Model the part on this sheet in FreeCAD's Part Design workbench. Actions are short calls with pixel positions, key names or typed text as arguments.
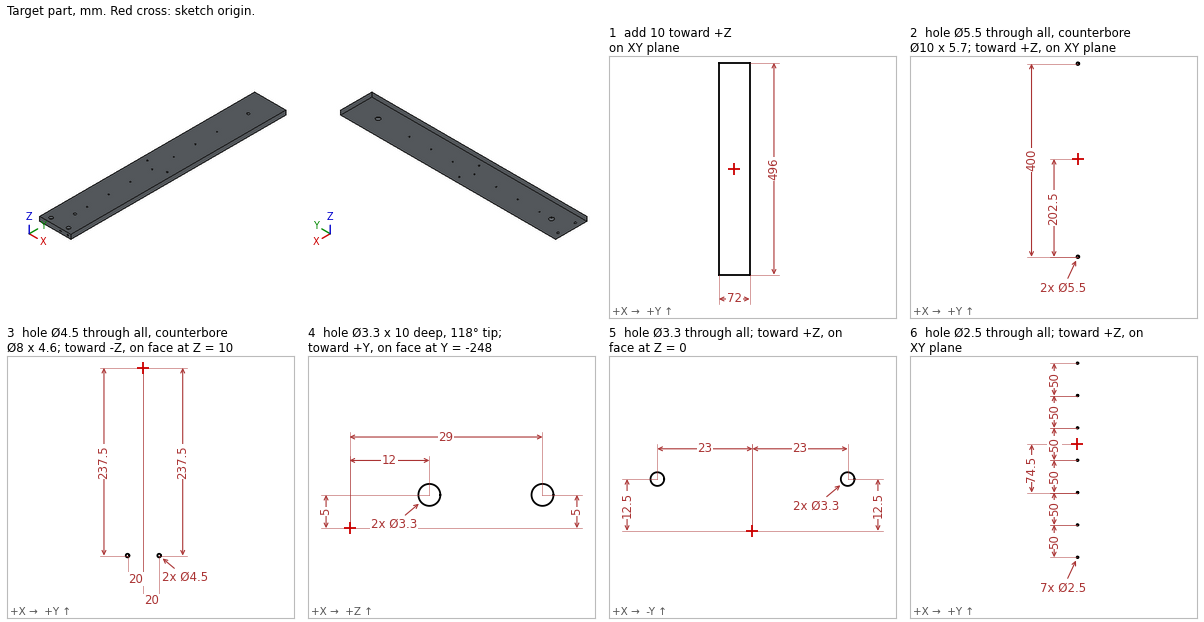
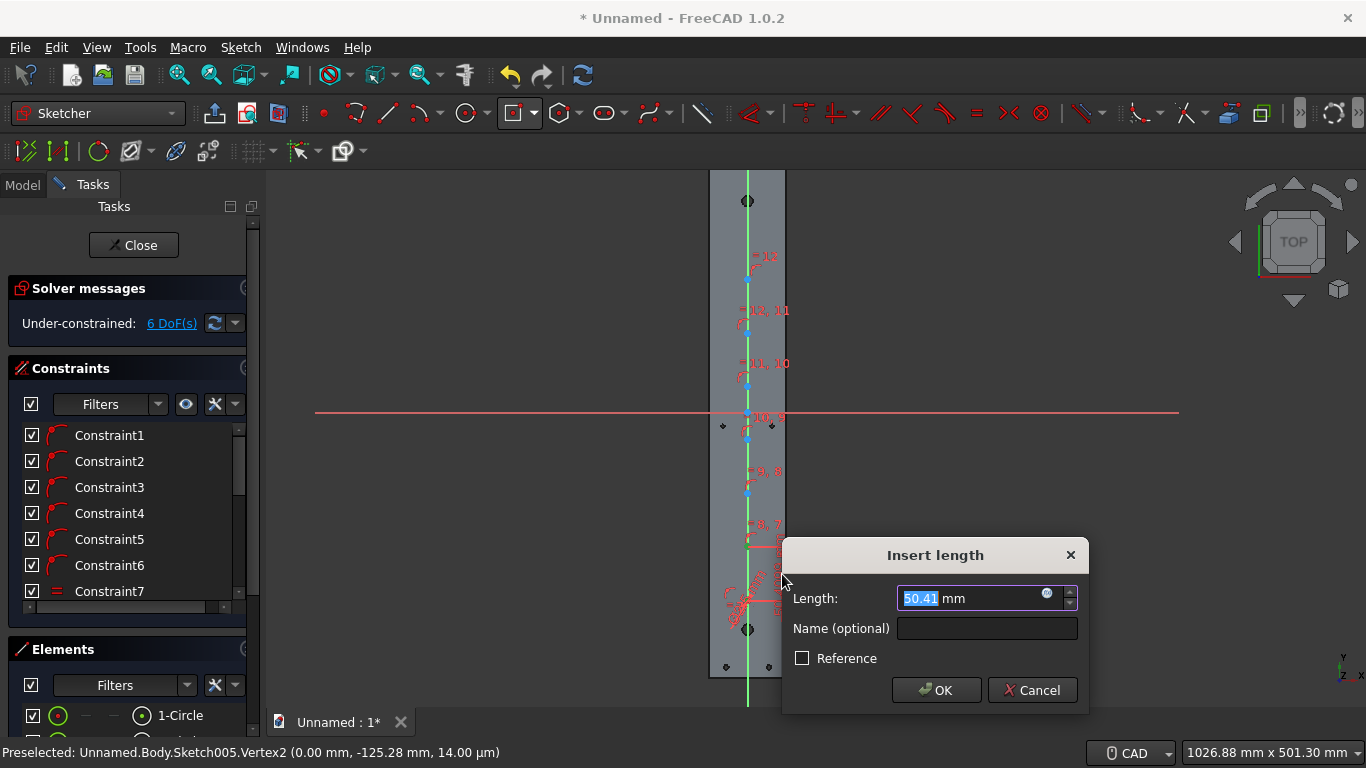
text(50)
key(Return)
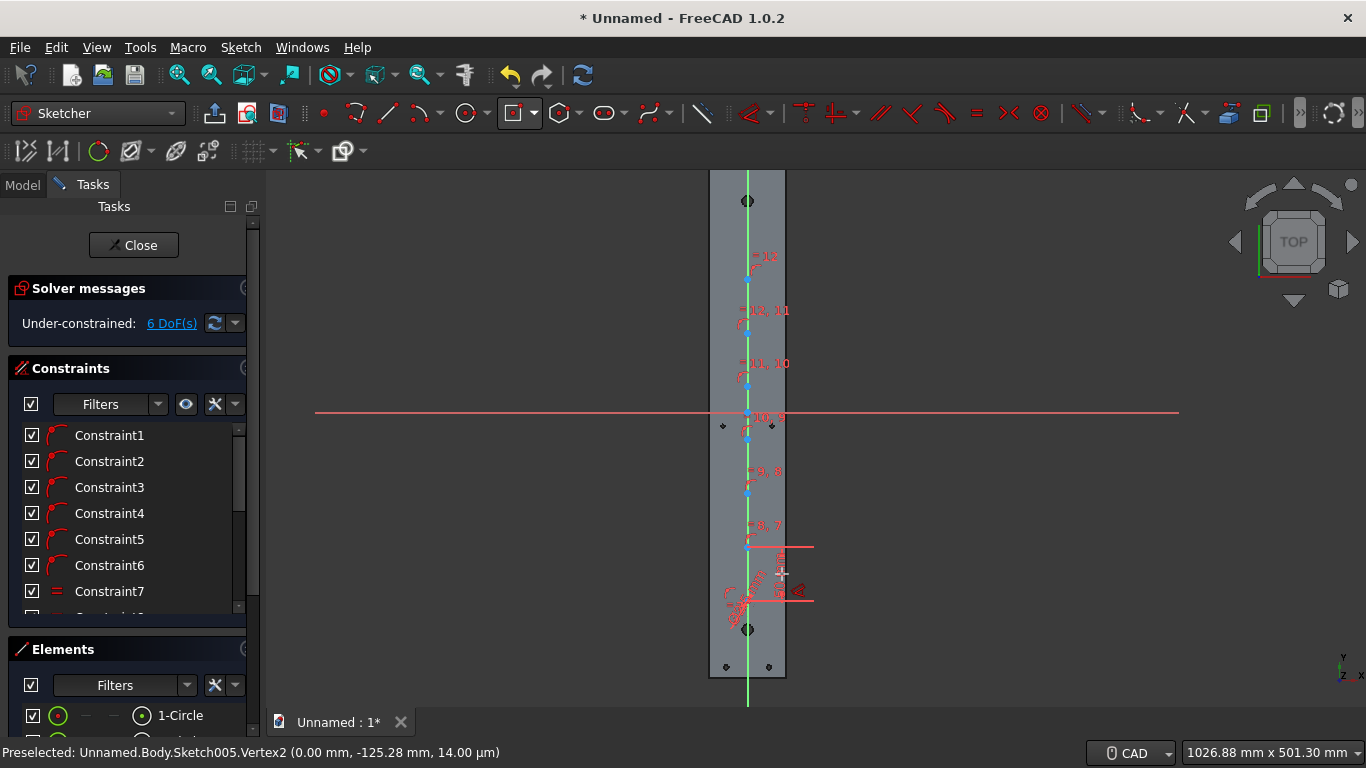
click(748, 547)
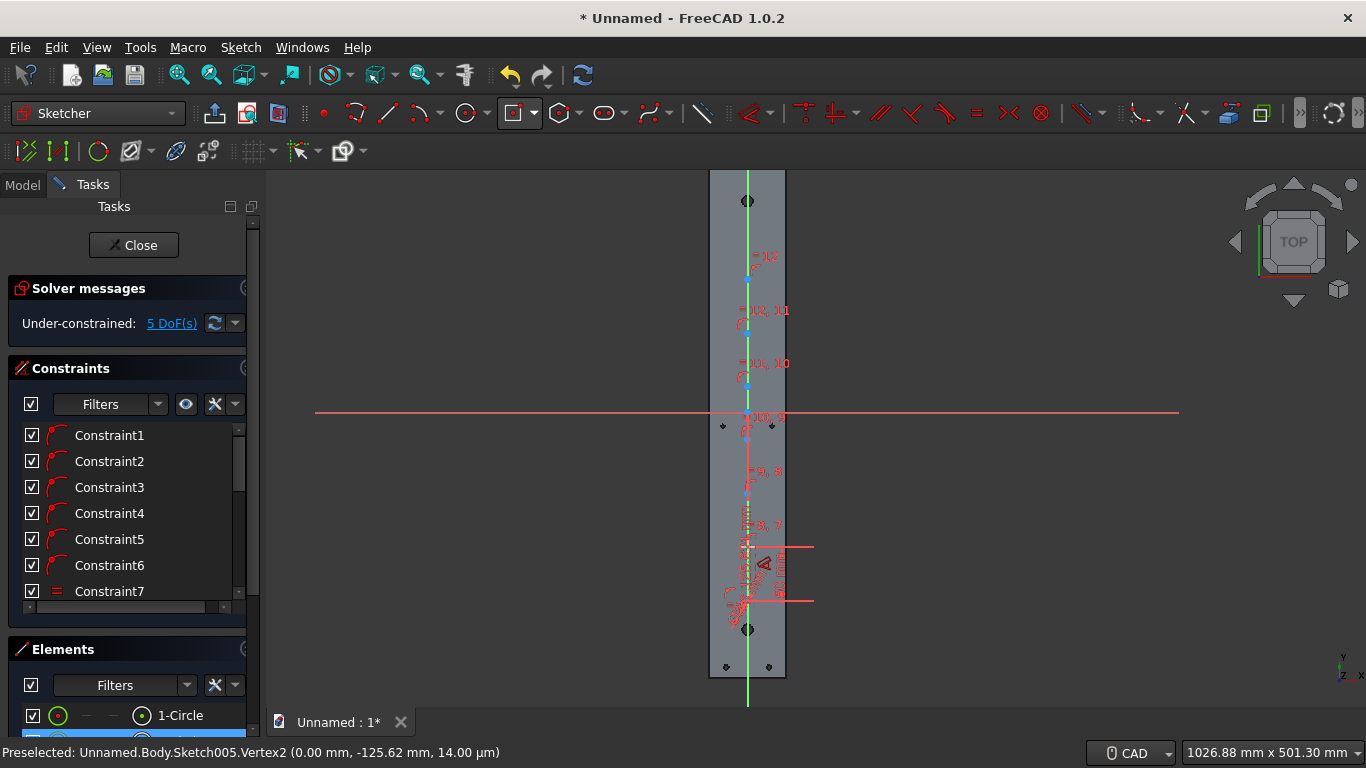
click(748, 494)
click(782, 521)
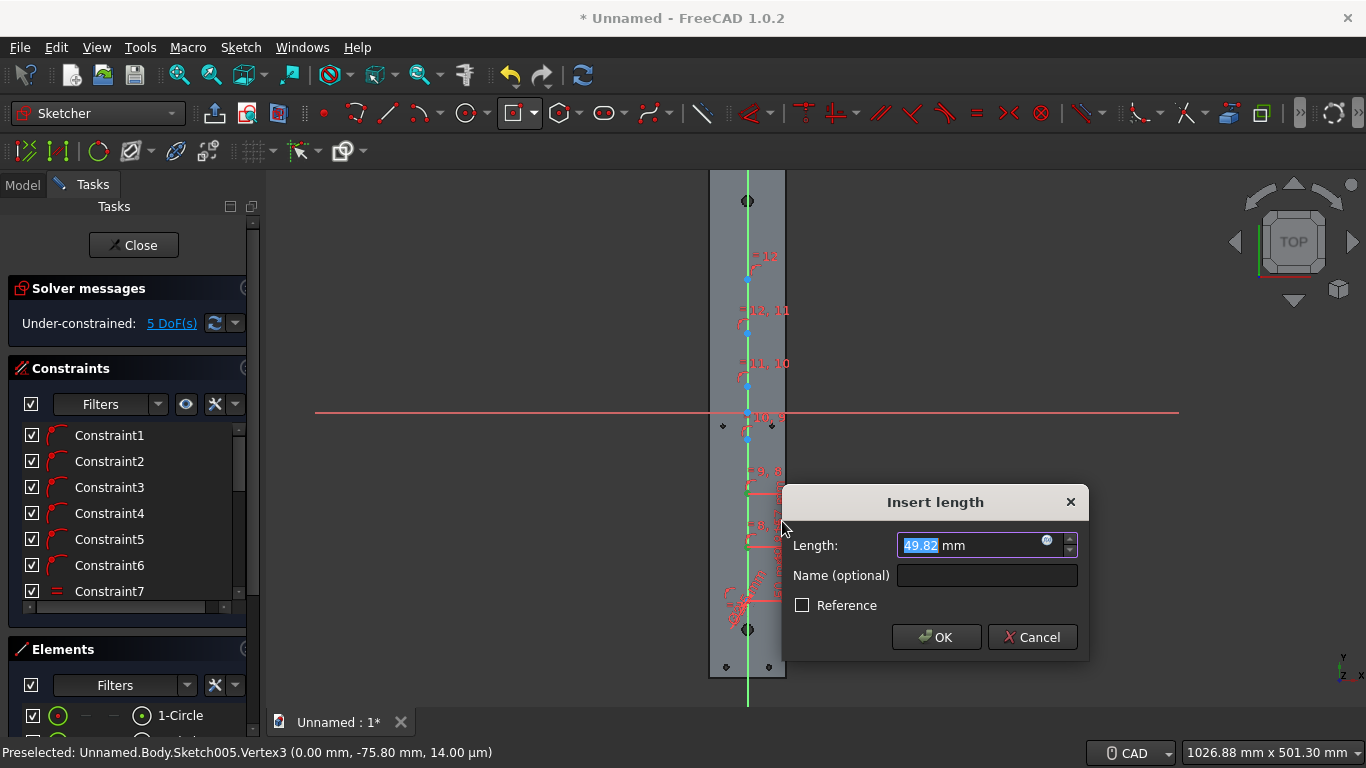
text(50)
key(Return)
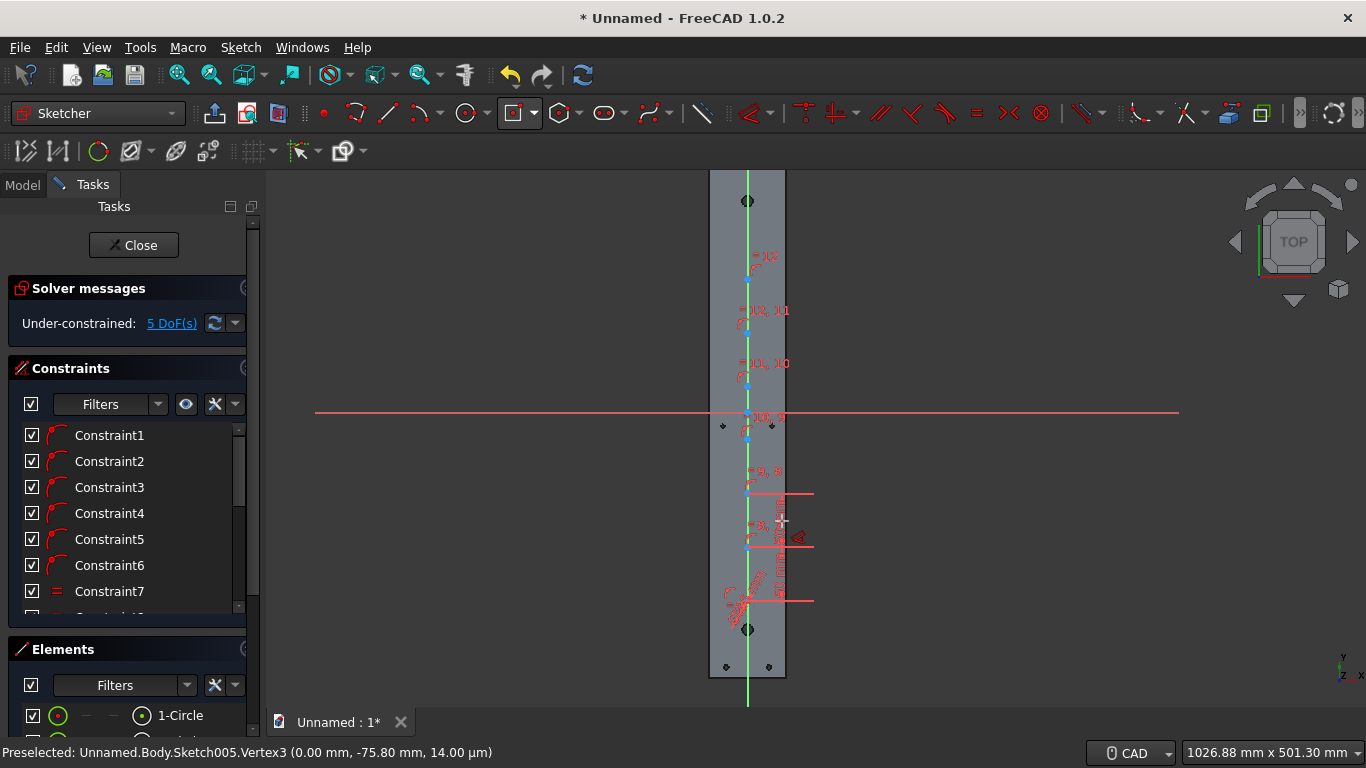
click(748, 494)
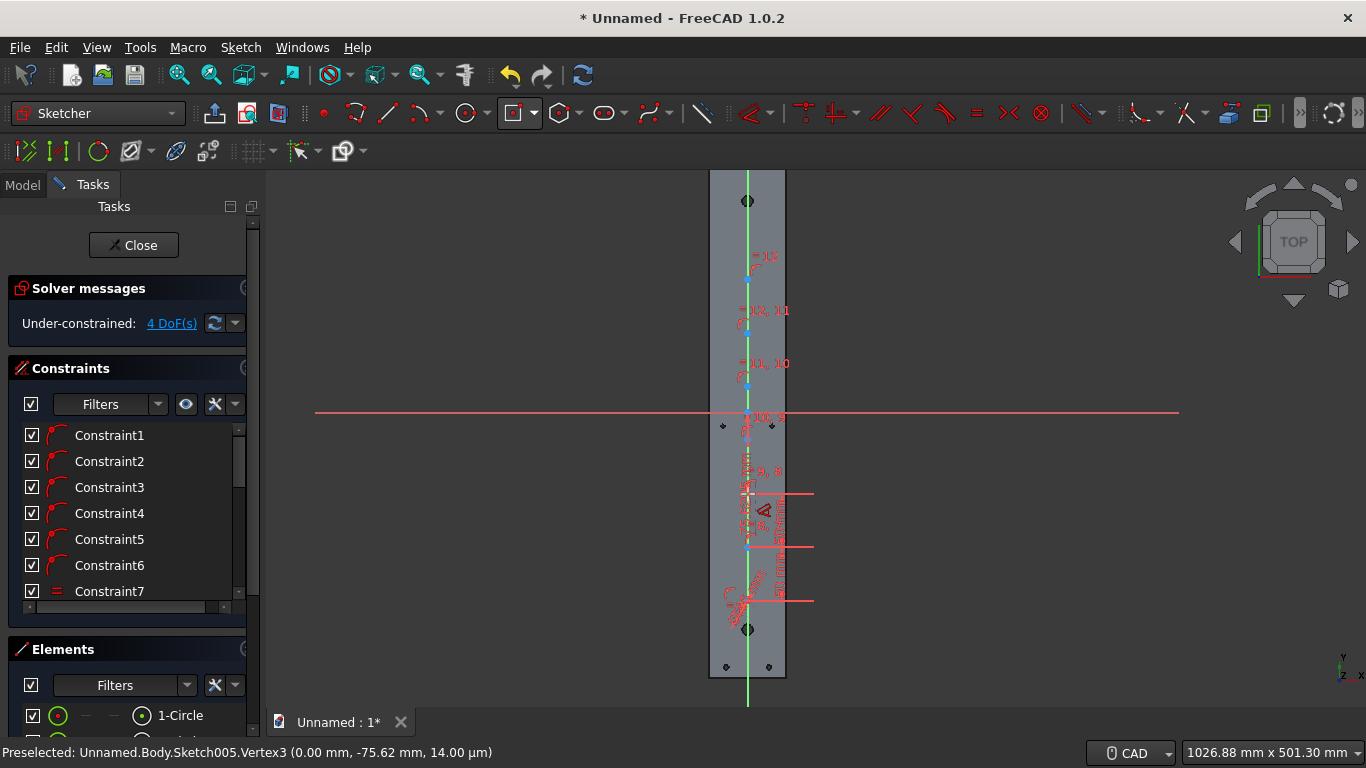
click(748, 440)
click(782, 467)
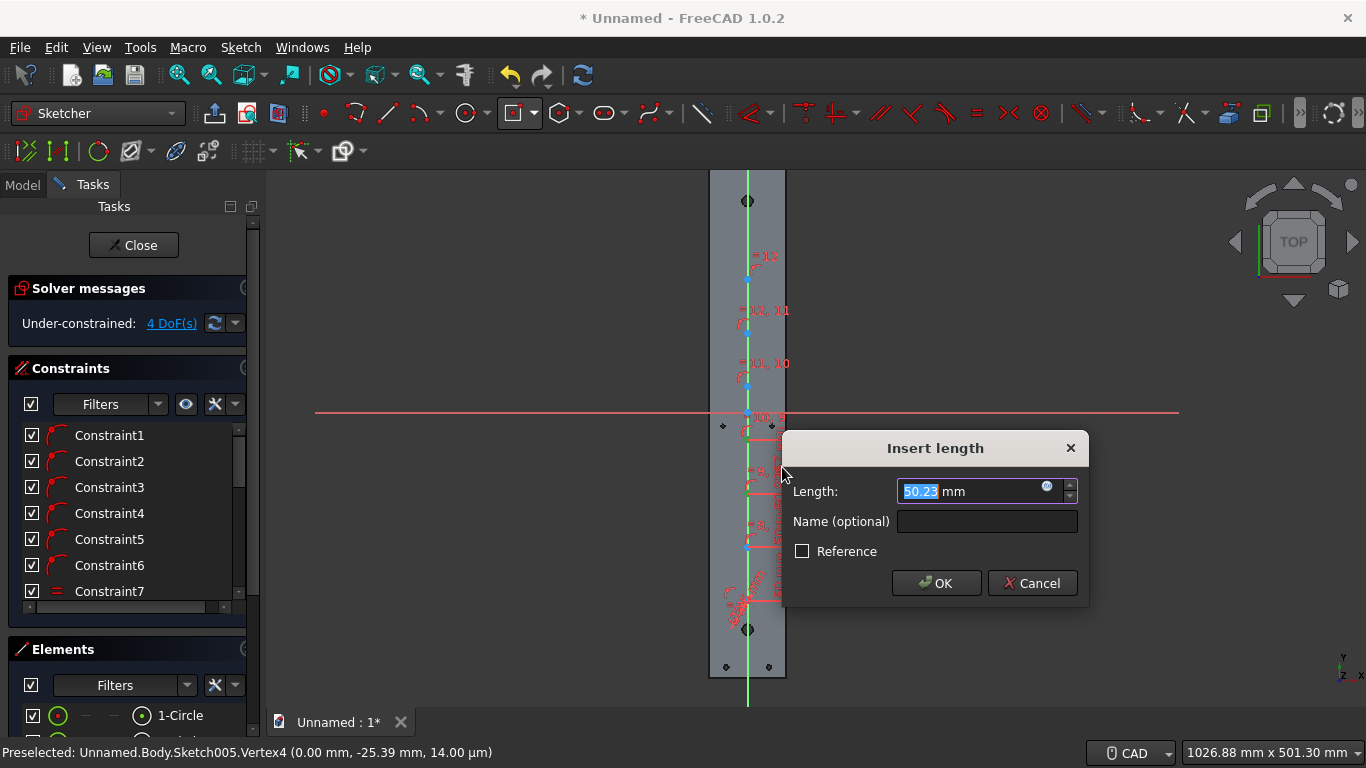
text(50)
key(Return)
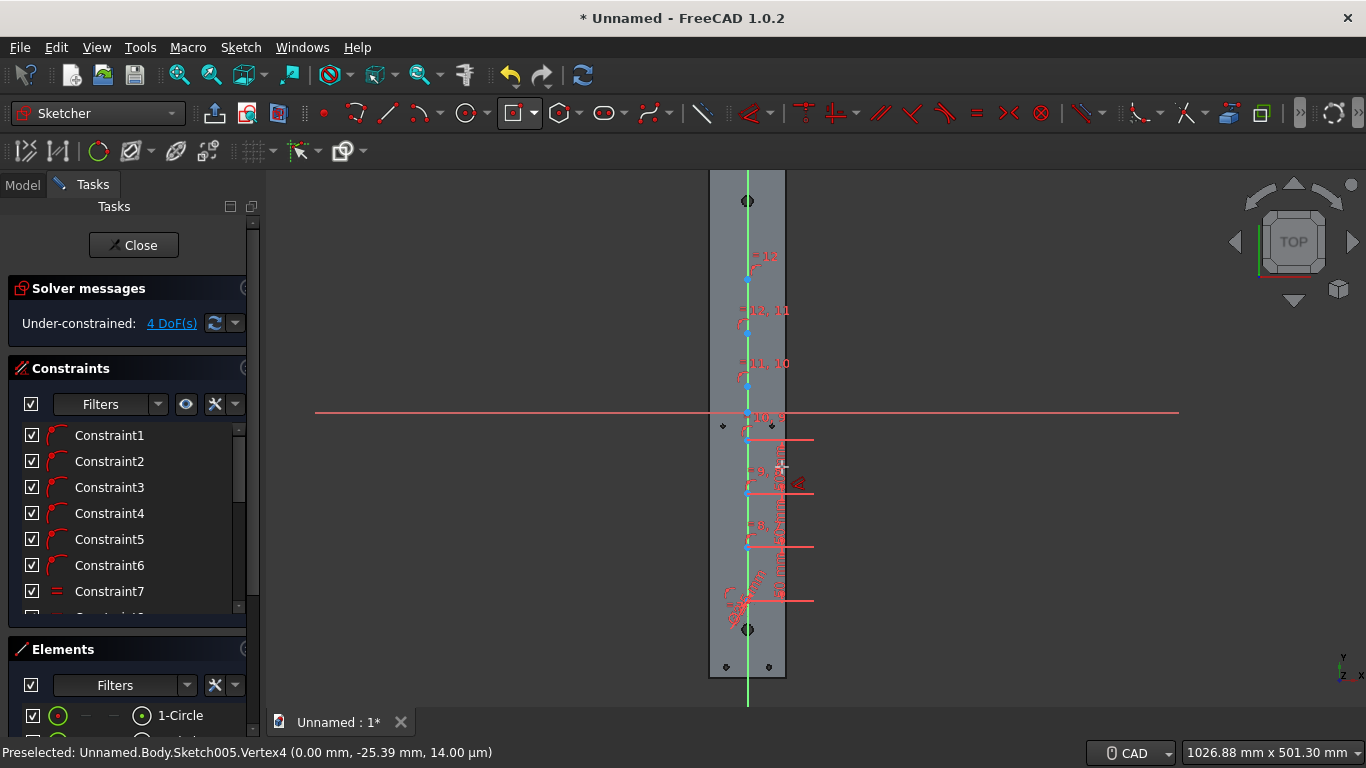
click(748, 440)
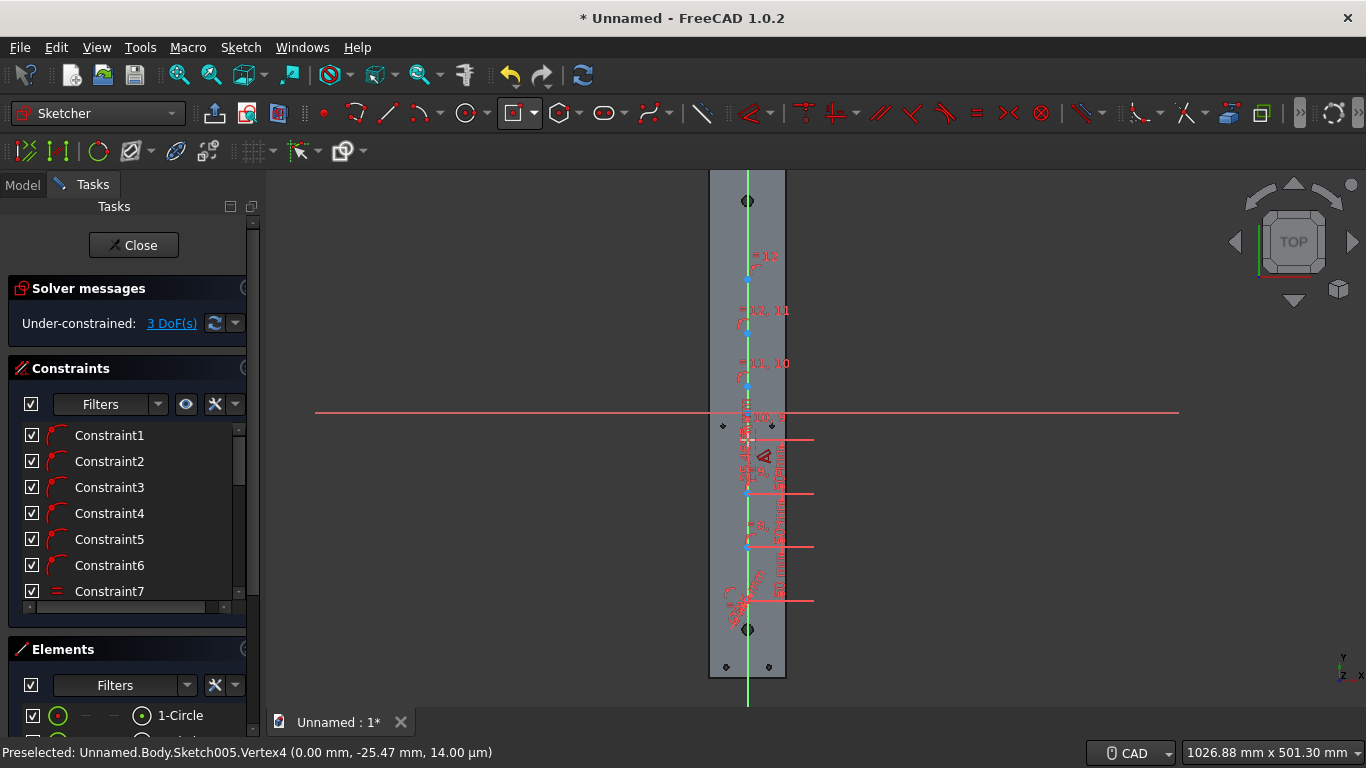
click(748, 386)
click(782, 394)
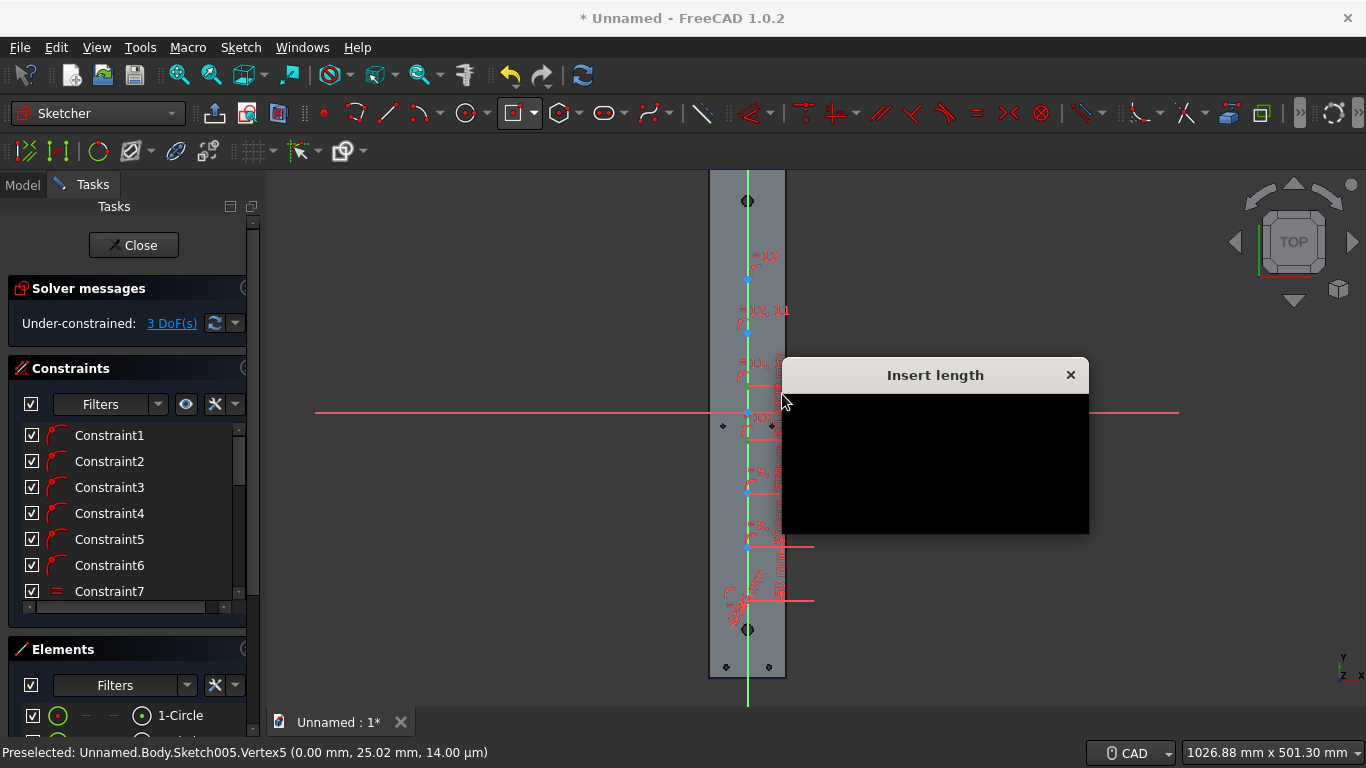
text(50)
key(Return)